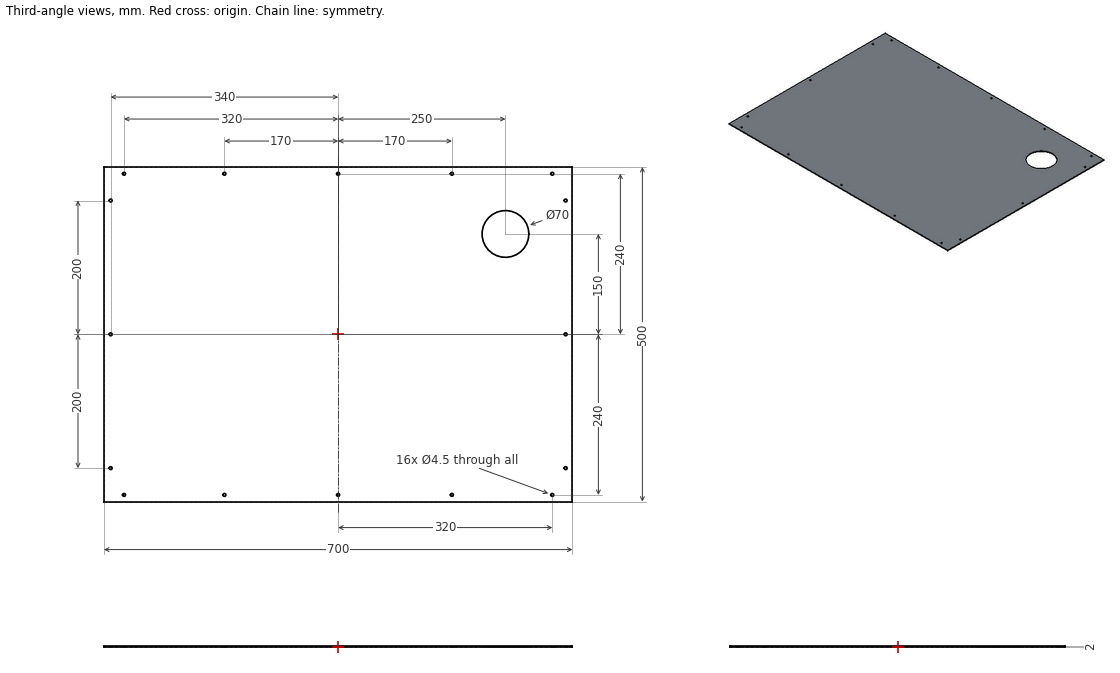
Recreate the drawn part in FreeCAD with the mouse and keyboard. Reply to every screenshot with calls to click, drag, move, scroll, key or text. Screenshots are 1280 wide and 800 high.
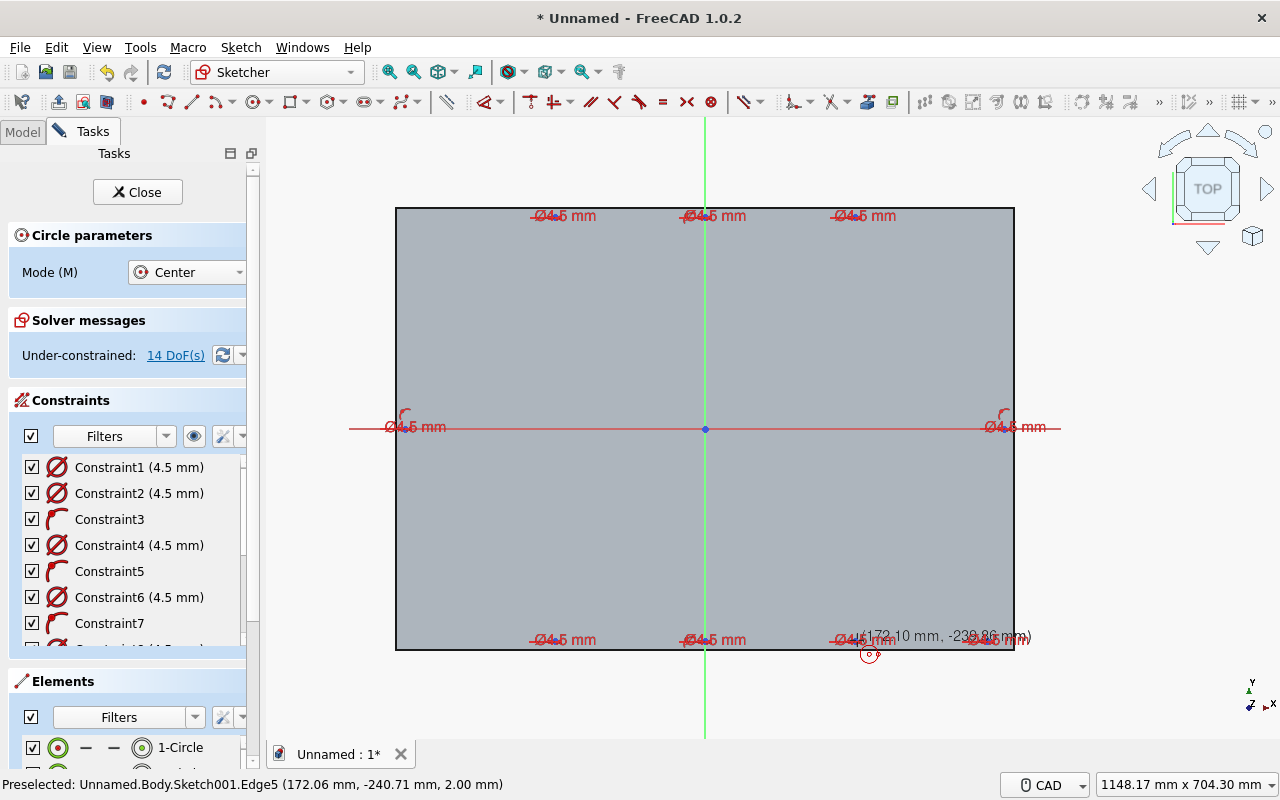
scroll(422, 217, up, 13)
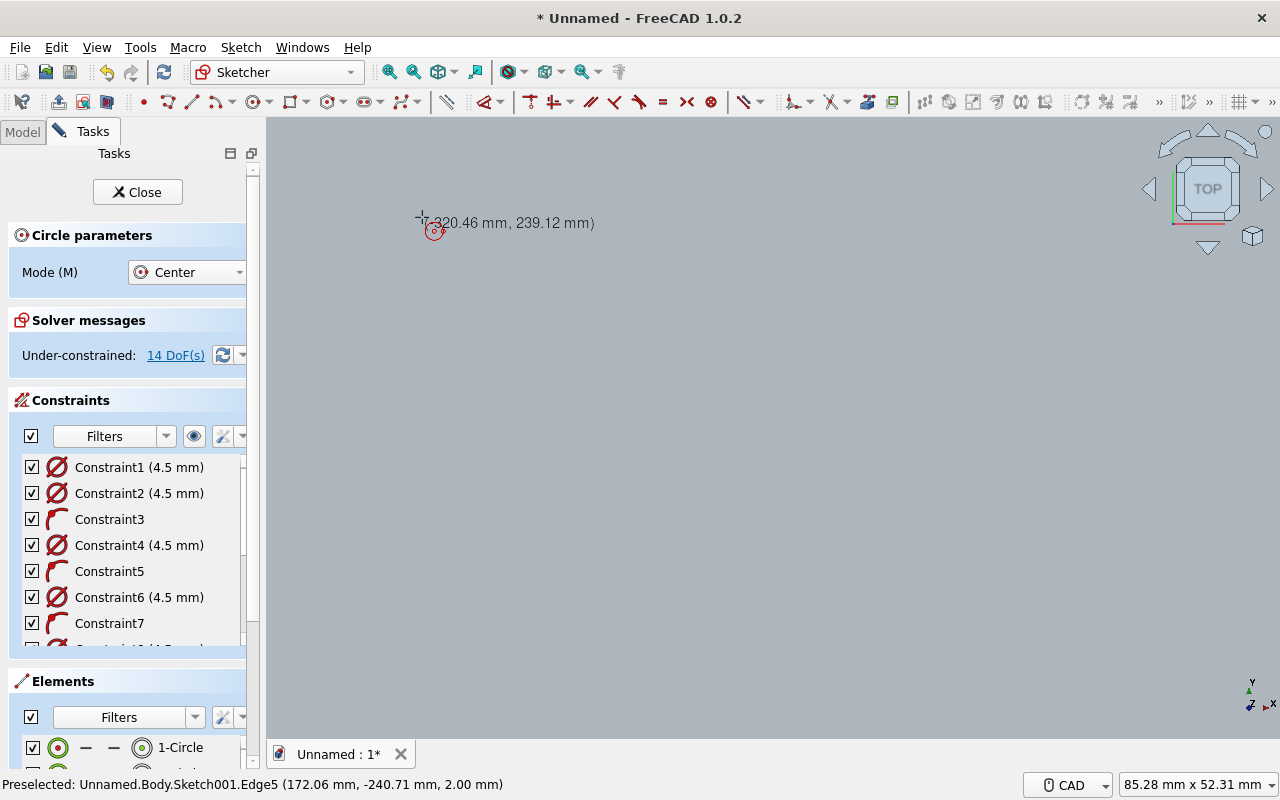
scroll(422, 216, down, 13)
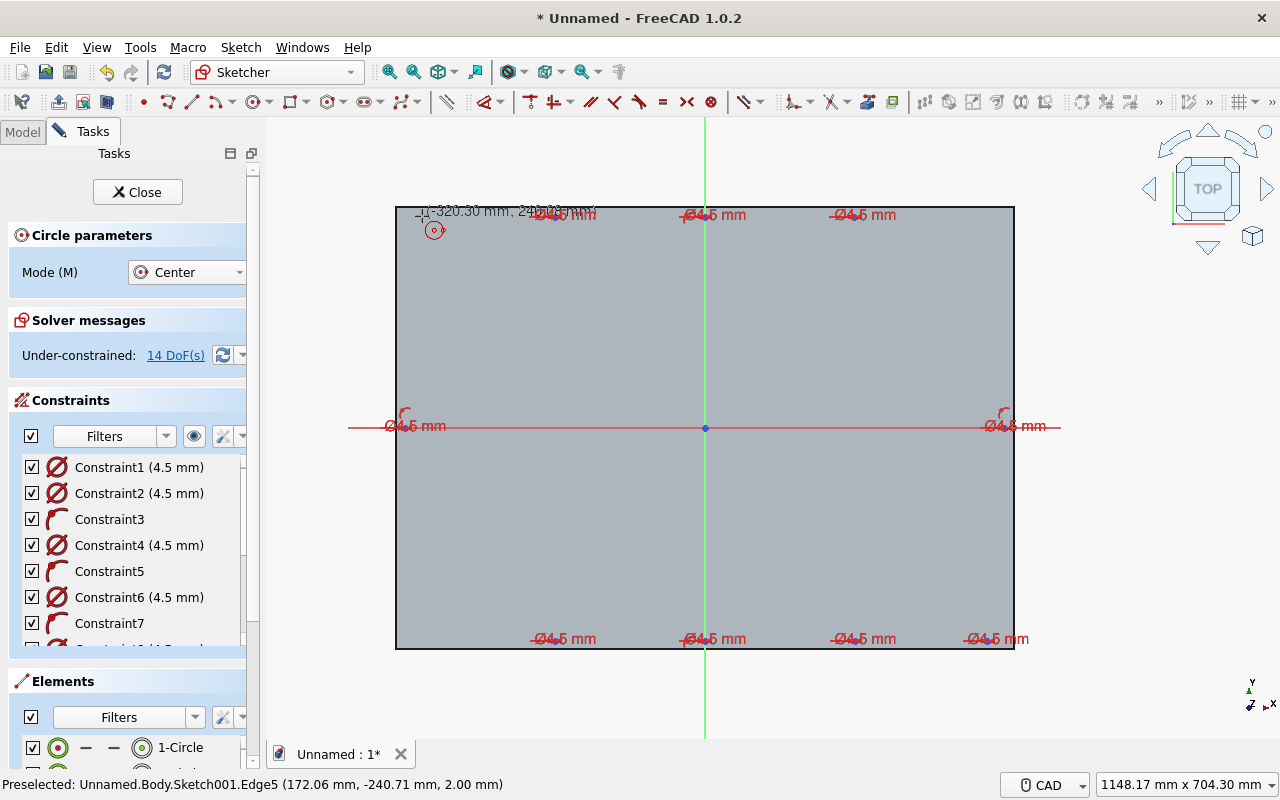
click(422, 216)
move(424, 215)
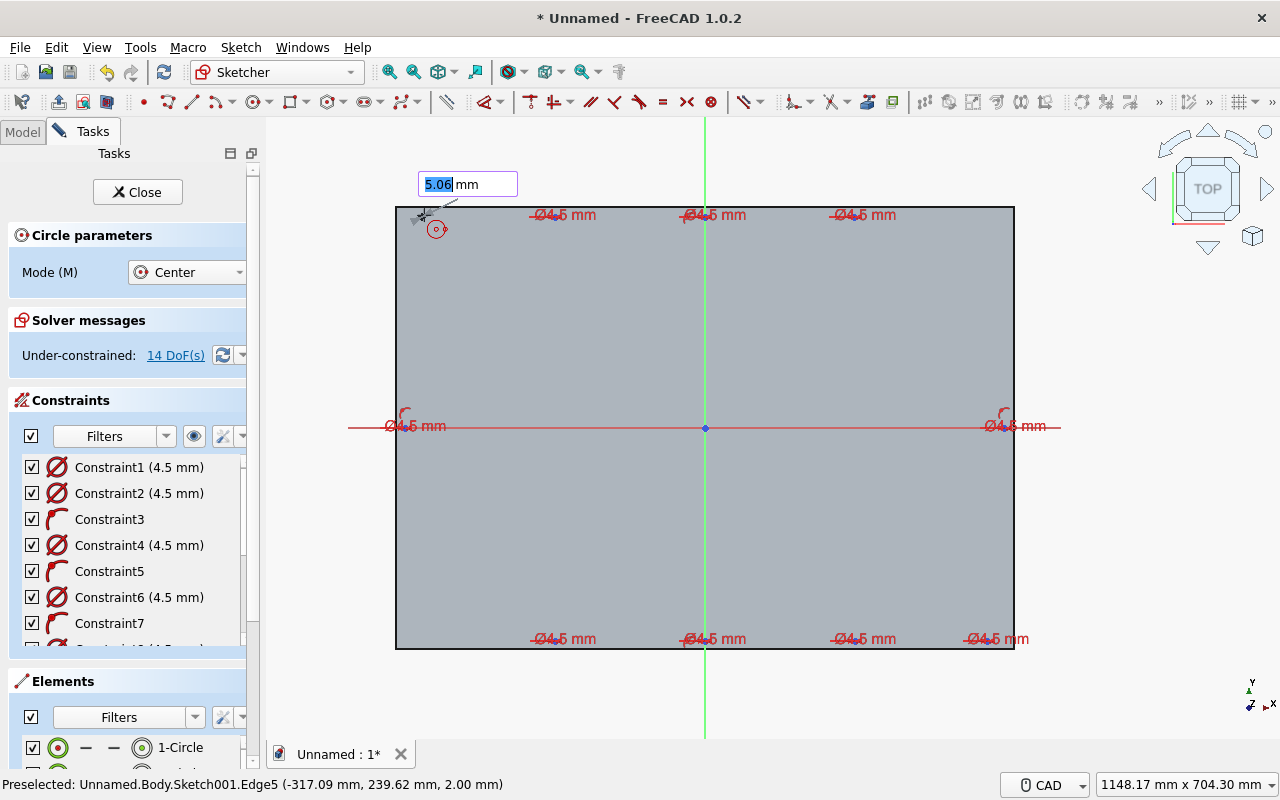
text(4.5)
key(Return)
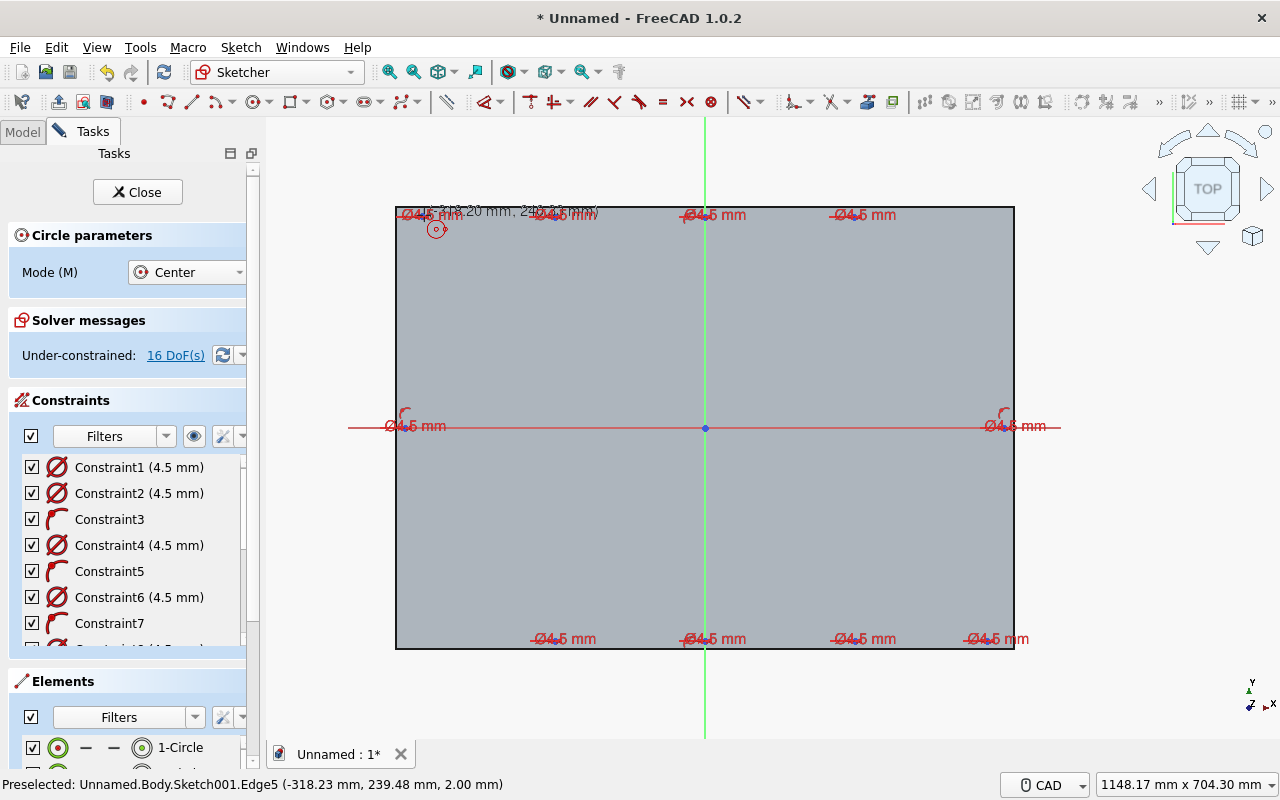
scroll(988, 216, up, 13)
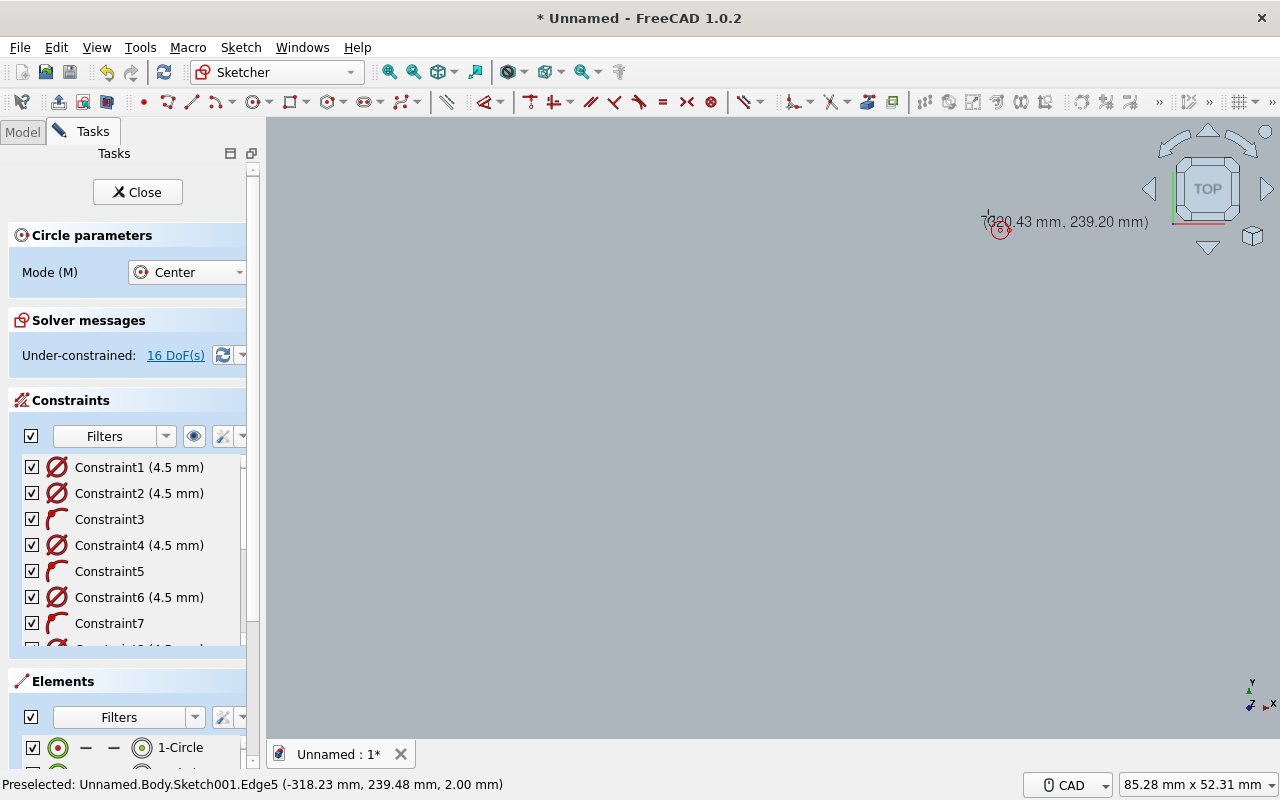
scroll(988, 216, down, 13)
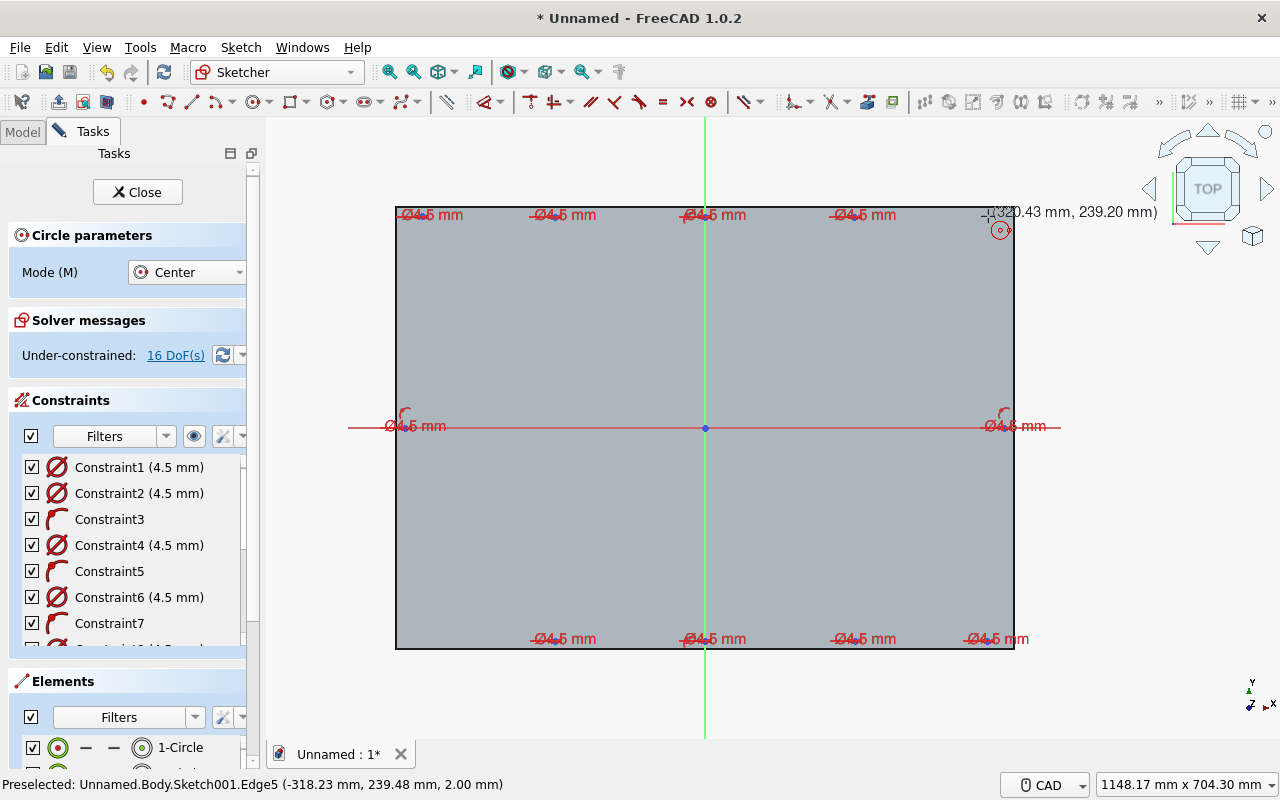
click(988, 216)
move(989, 215)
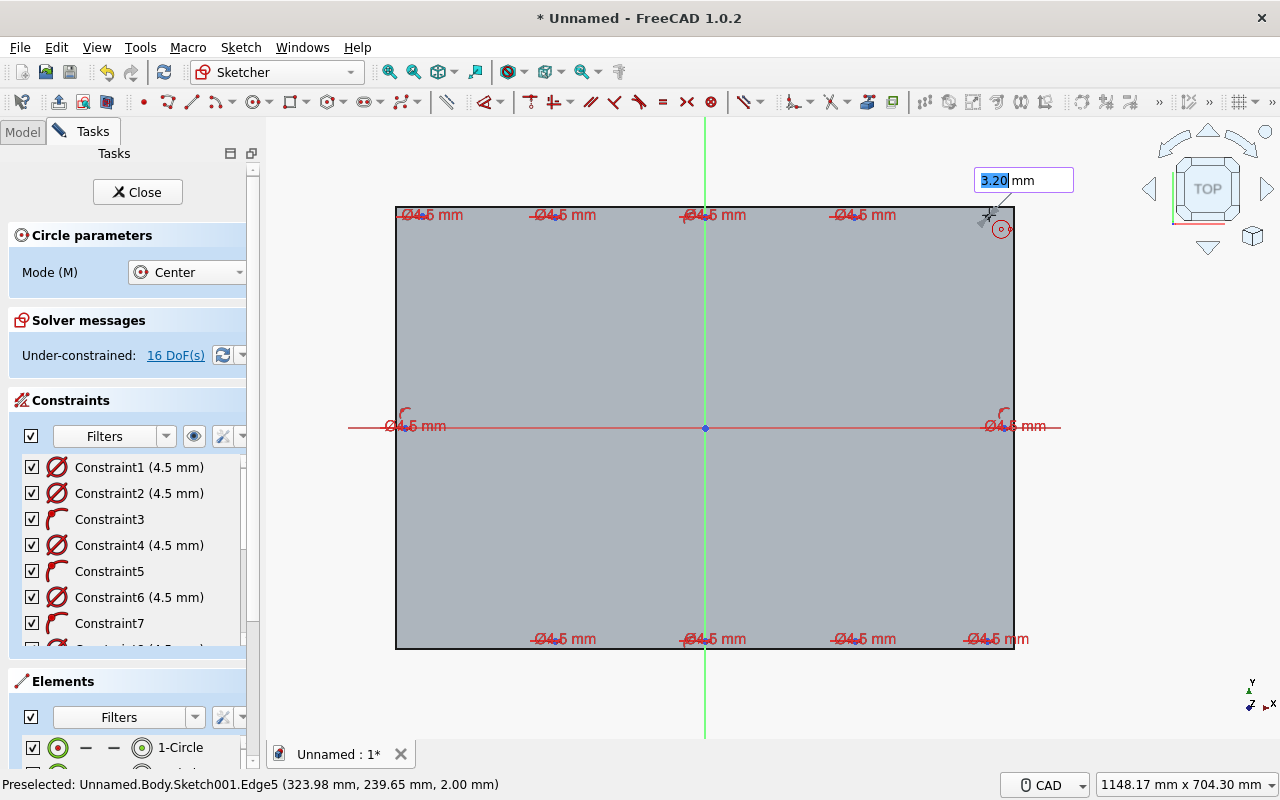
text(4.5)
key(Return)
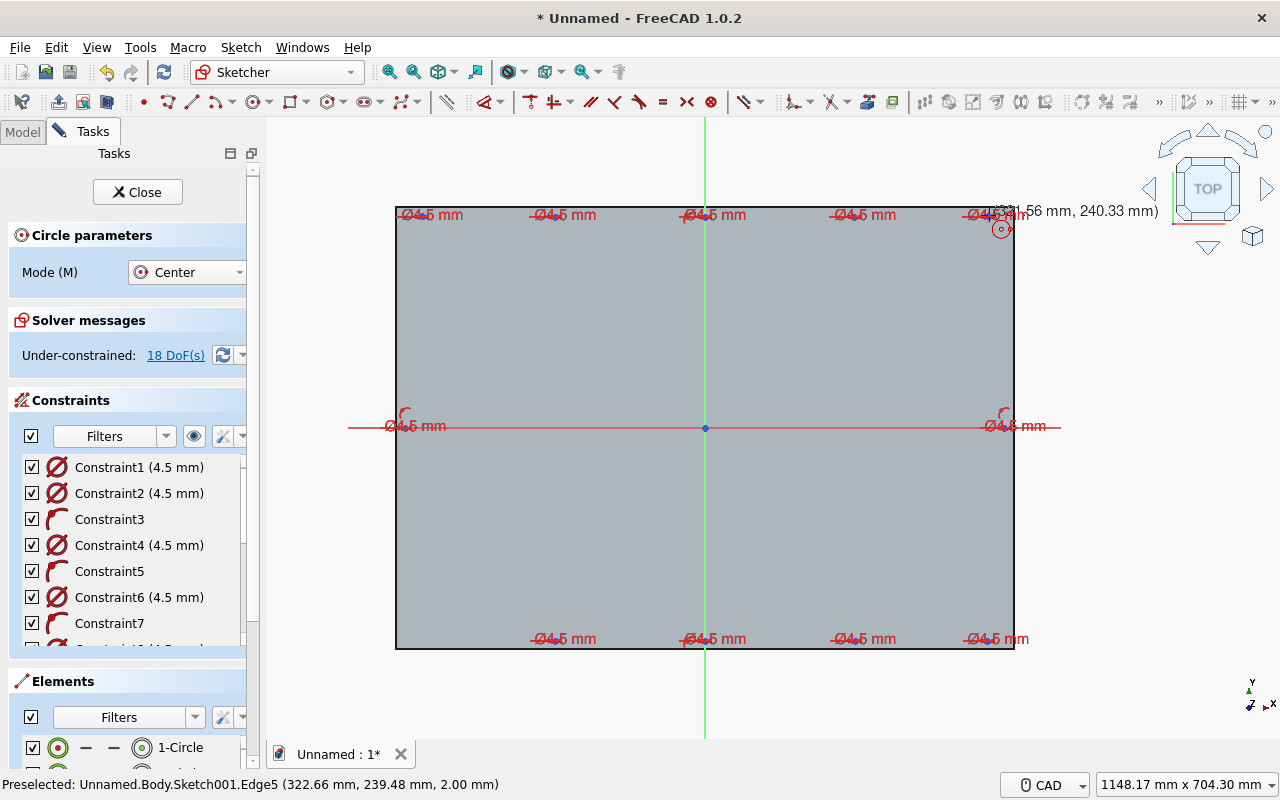
scroll(405, 252, up, 13)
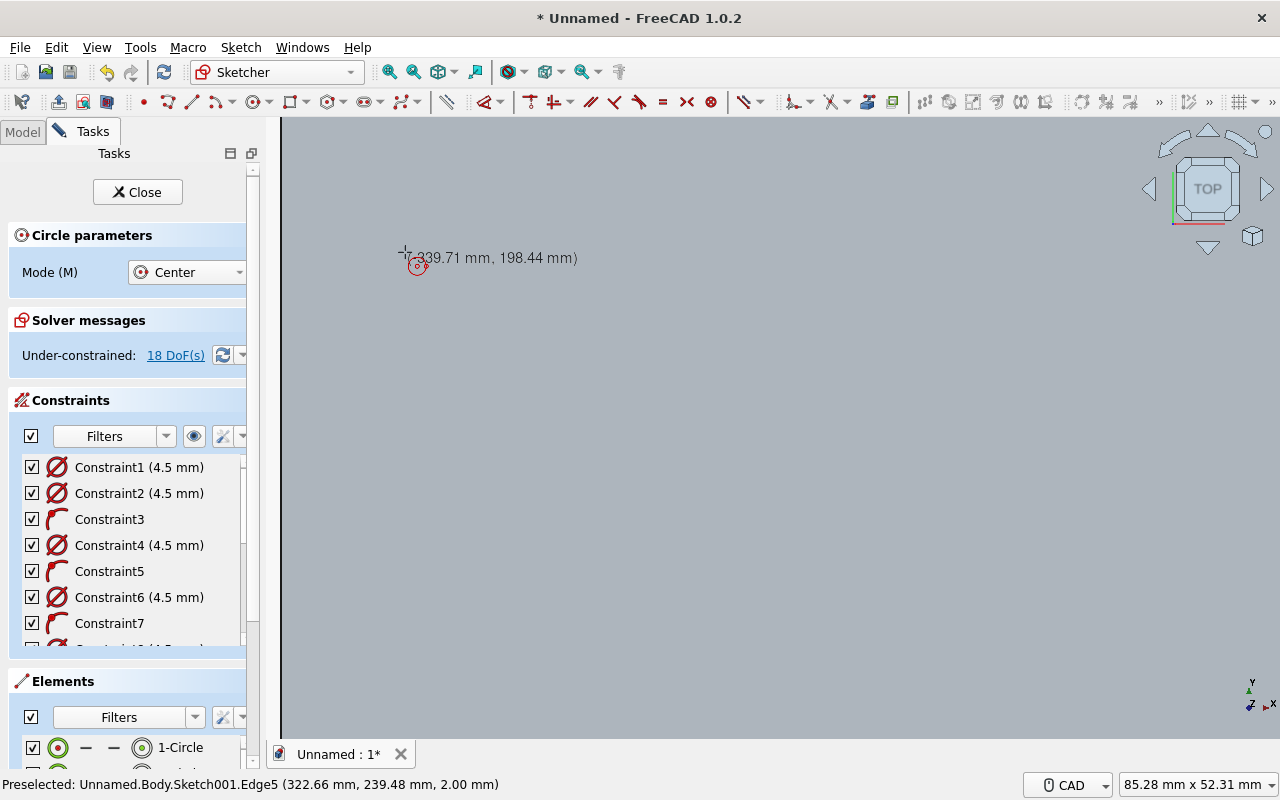
scroll(405, 252, down, 13)